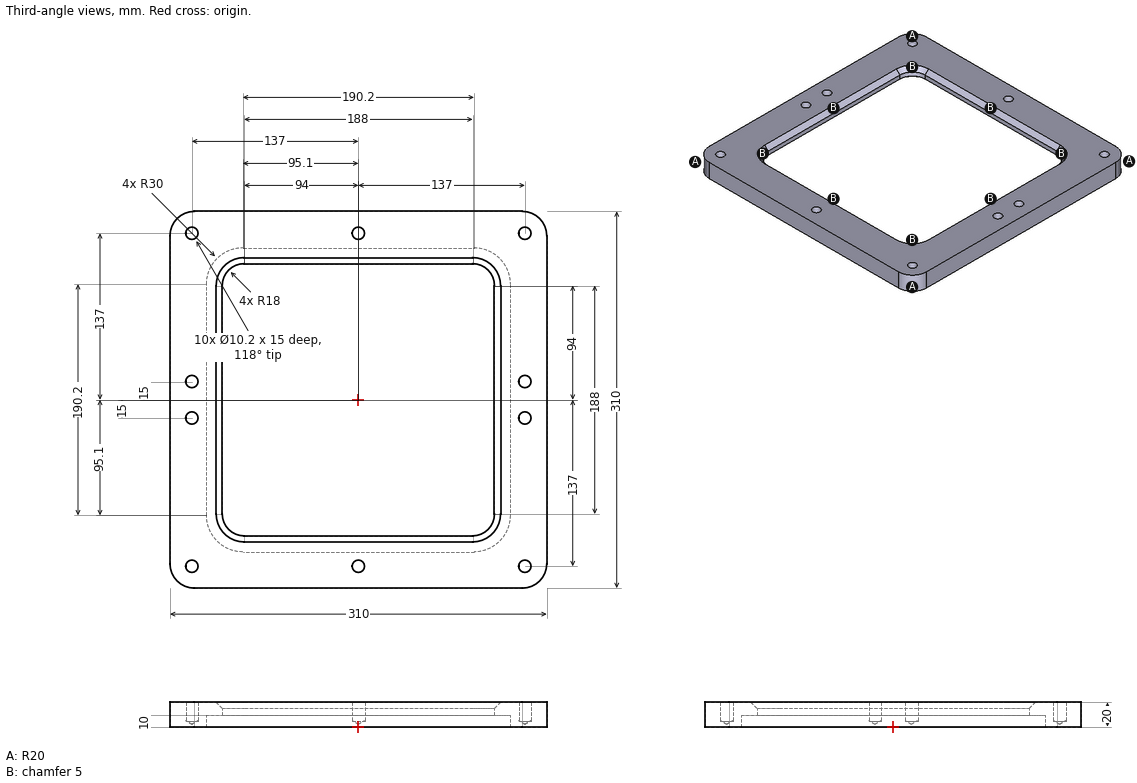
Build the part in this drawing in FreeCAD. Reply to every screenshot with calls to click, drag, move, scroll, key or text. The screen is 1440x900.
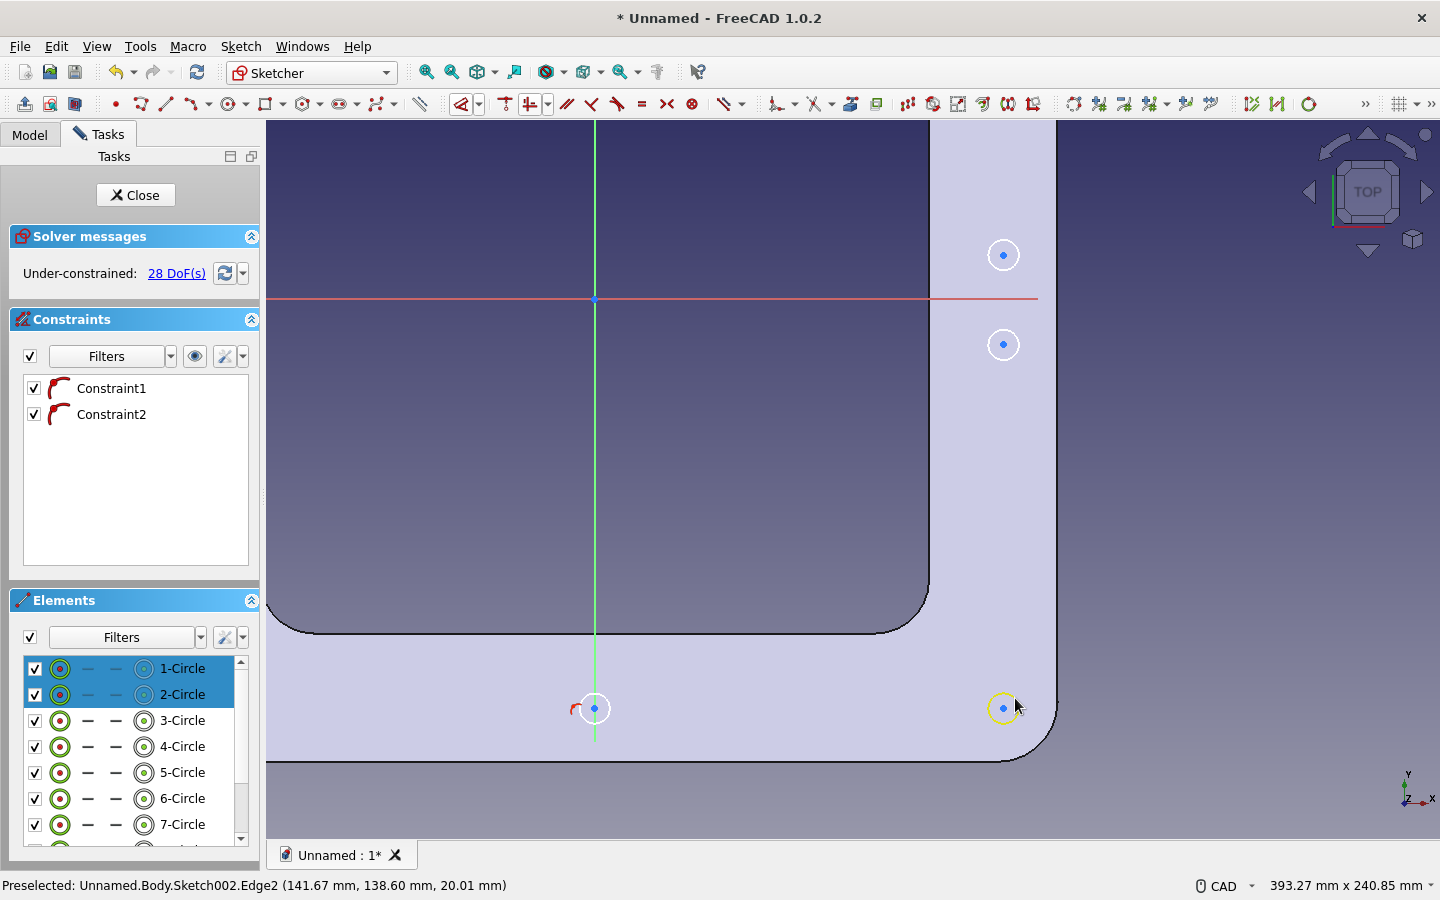
click(1014, 698)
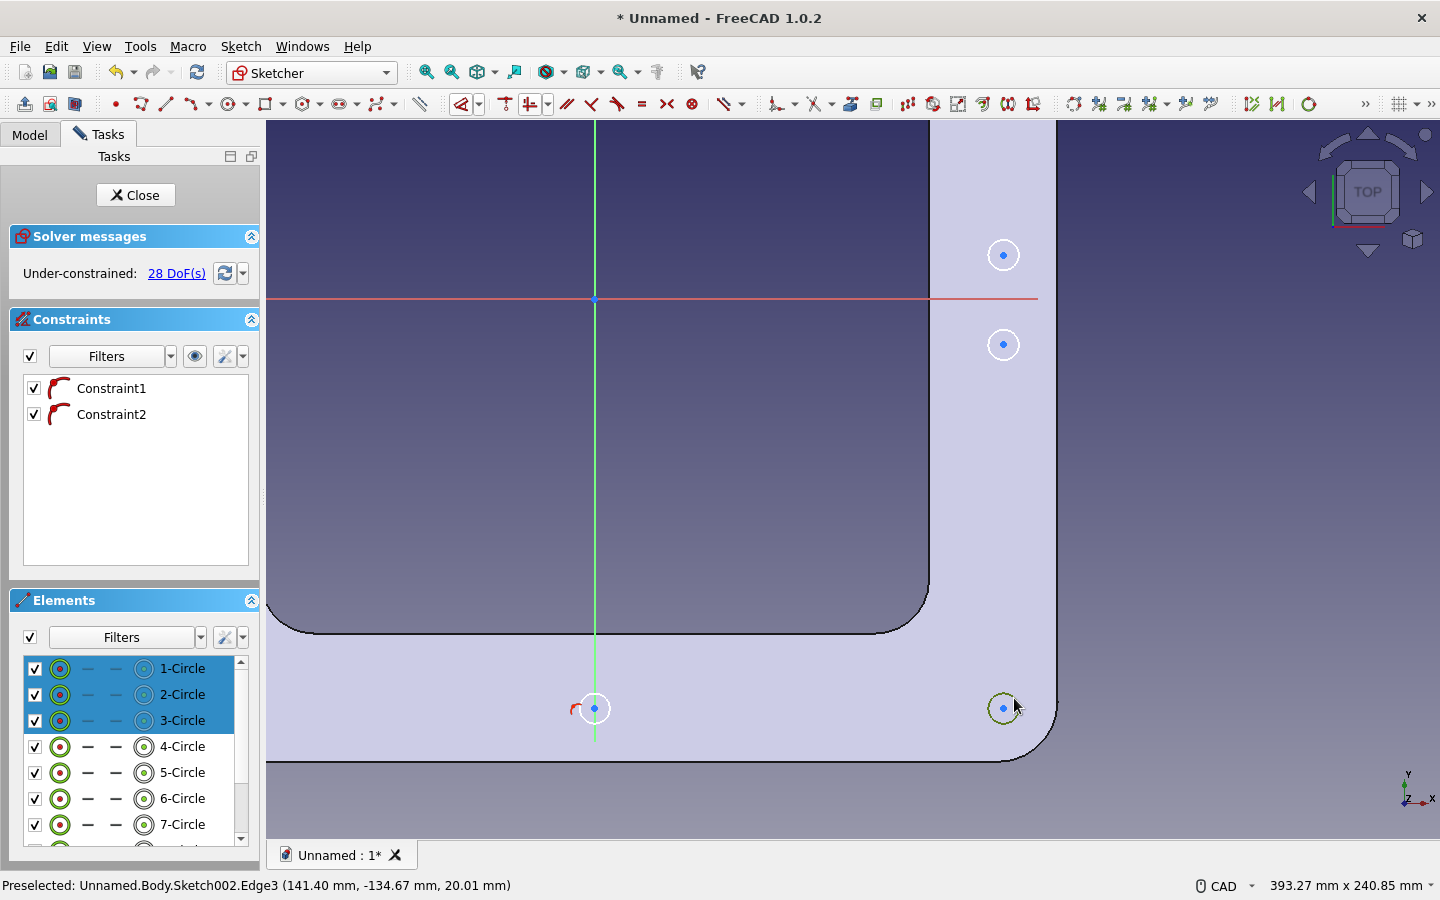
scroll(1015, 699, down, 3)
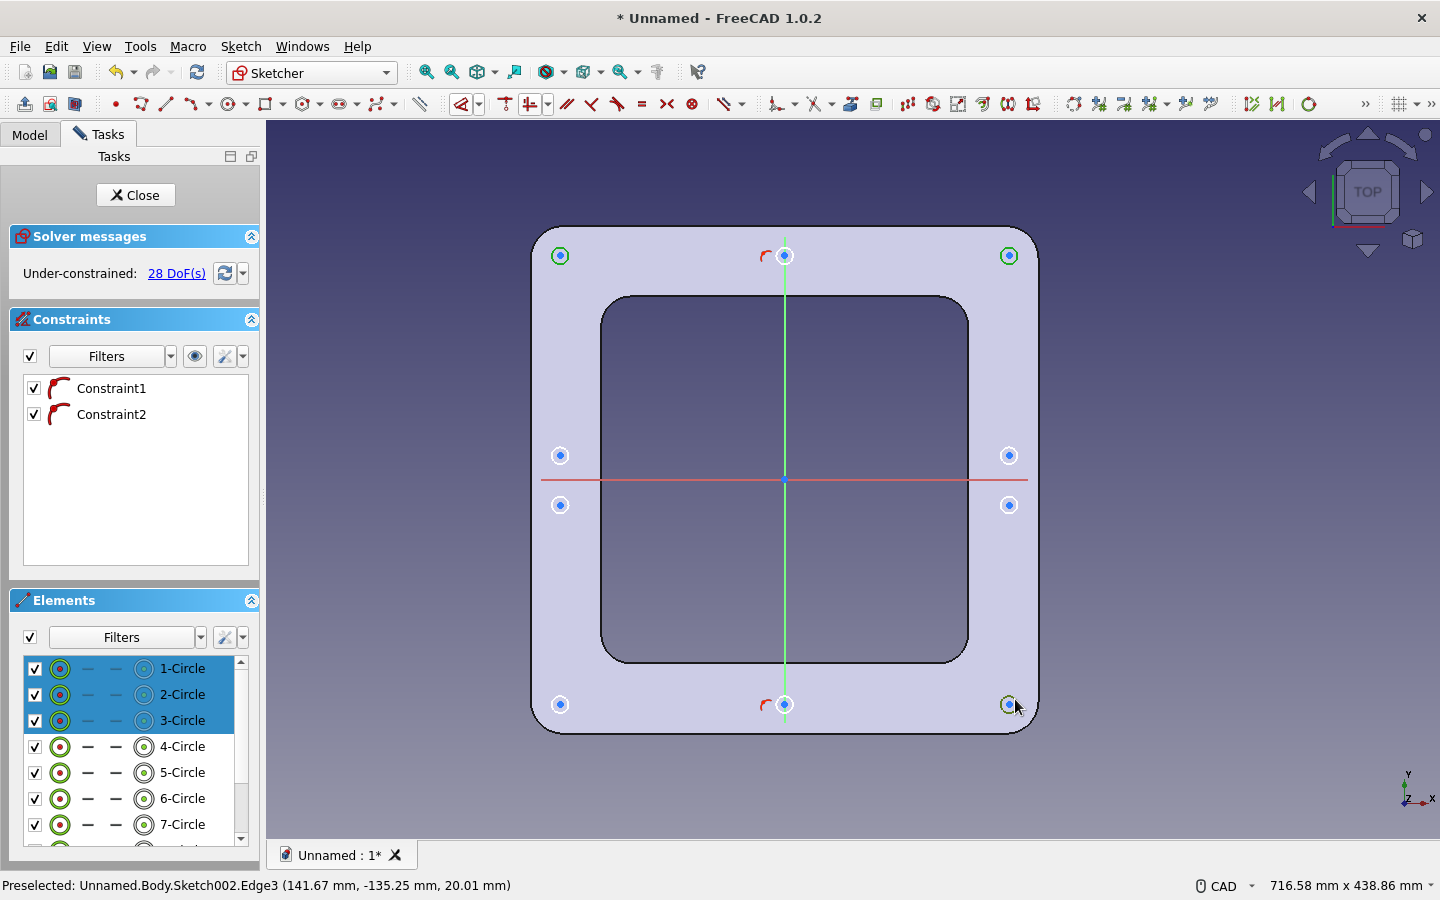
scroll(566, 699, up, 3)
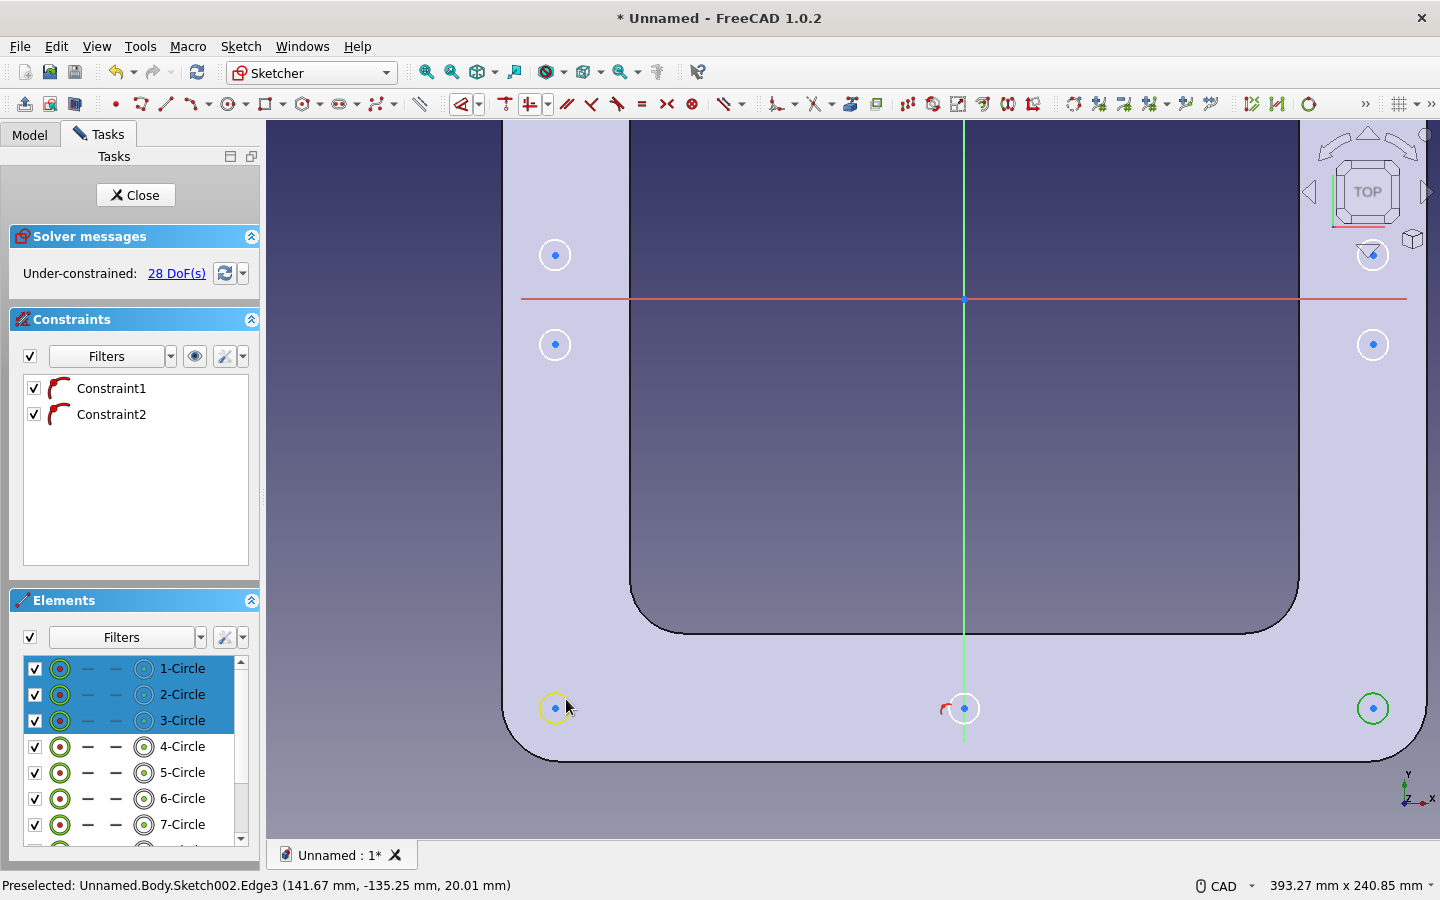
click(566, 698)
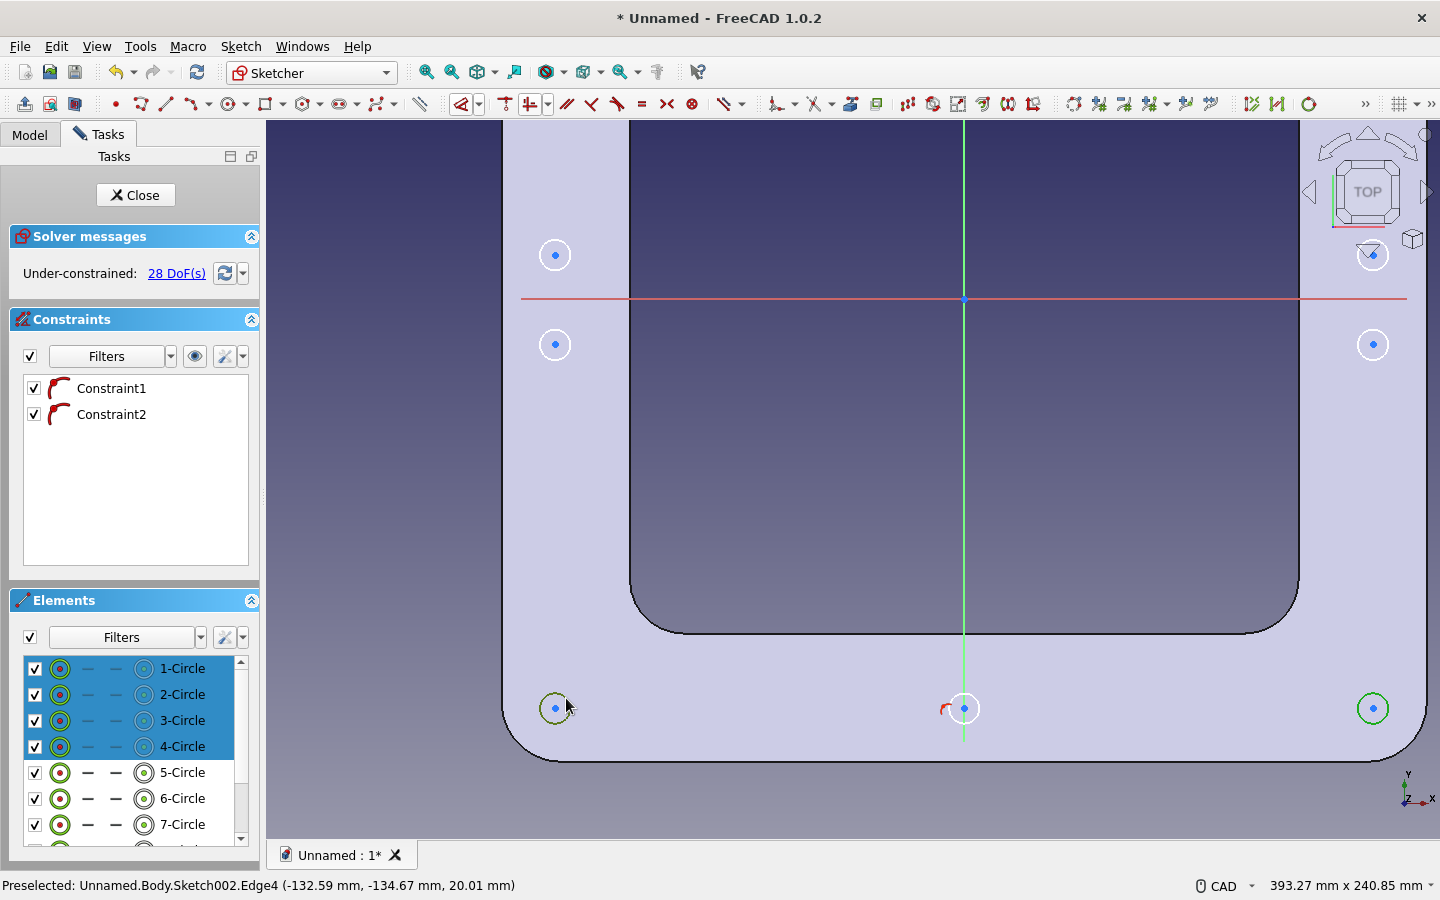
scroll(975, 698, up, 2)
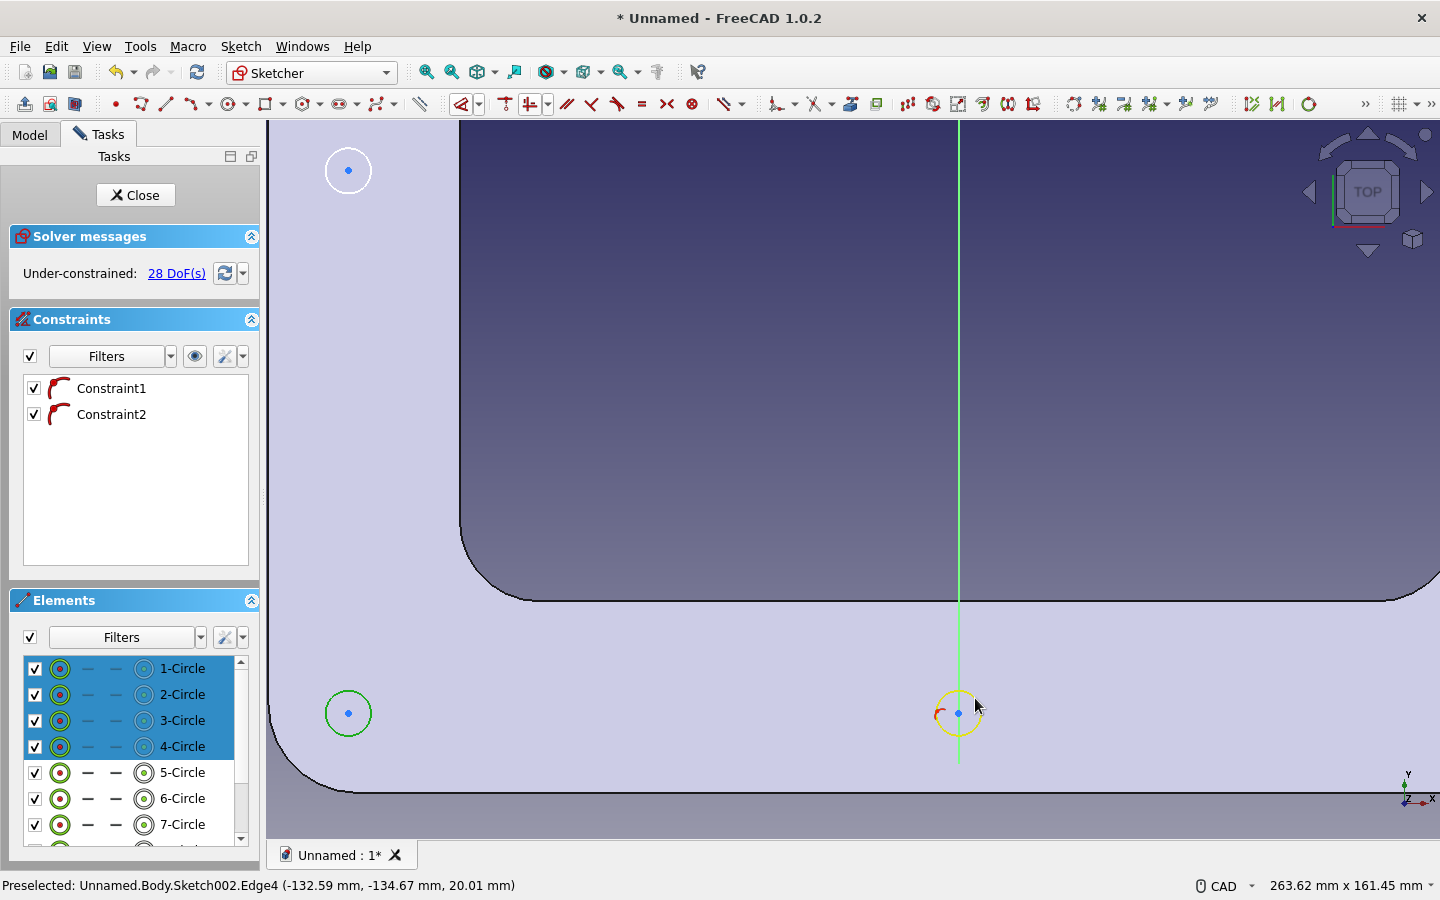
click(974, 697)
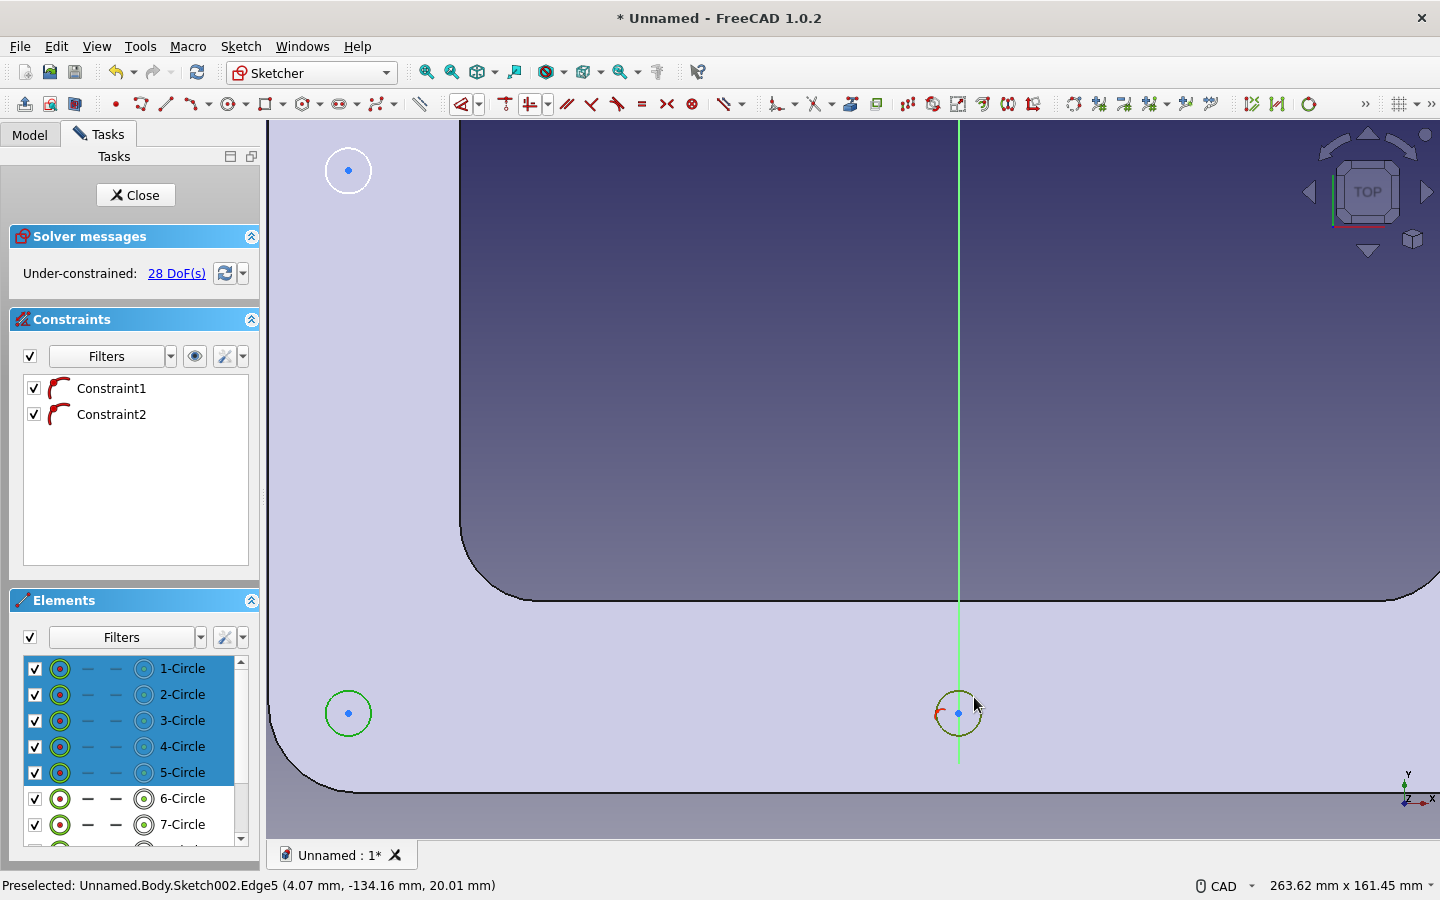
scroll(683, 699, down, 5)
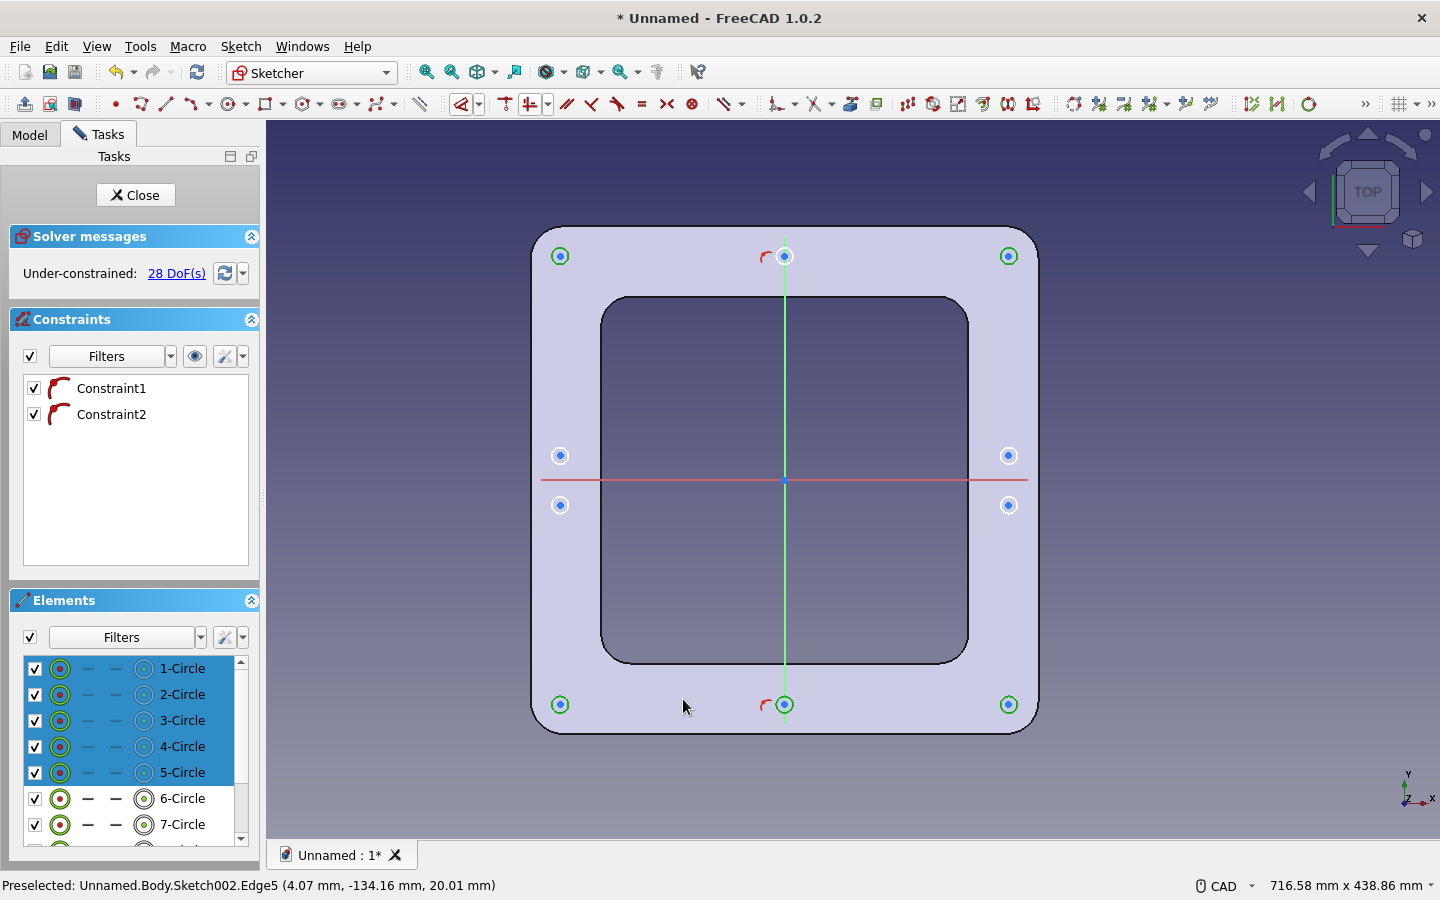
scroll(790, 250, up, 5)